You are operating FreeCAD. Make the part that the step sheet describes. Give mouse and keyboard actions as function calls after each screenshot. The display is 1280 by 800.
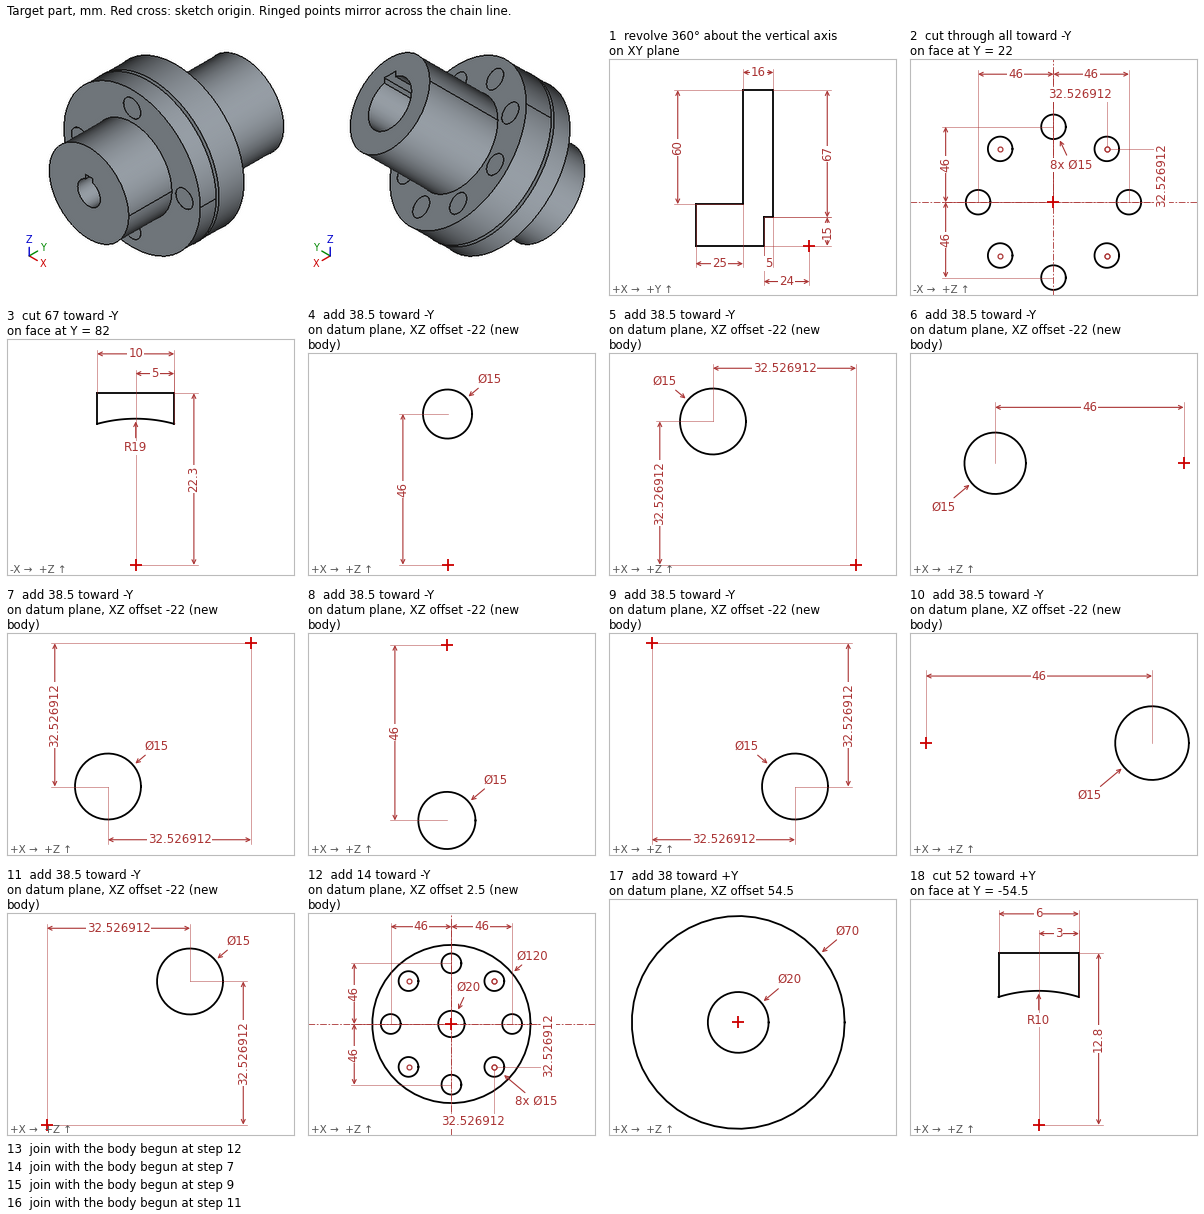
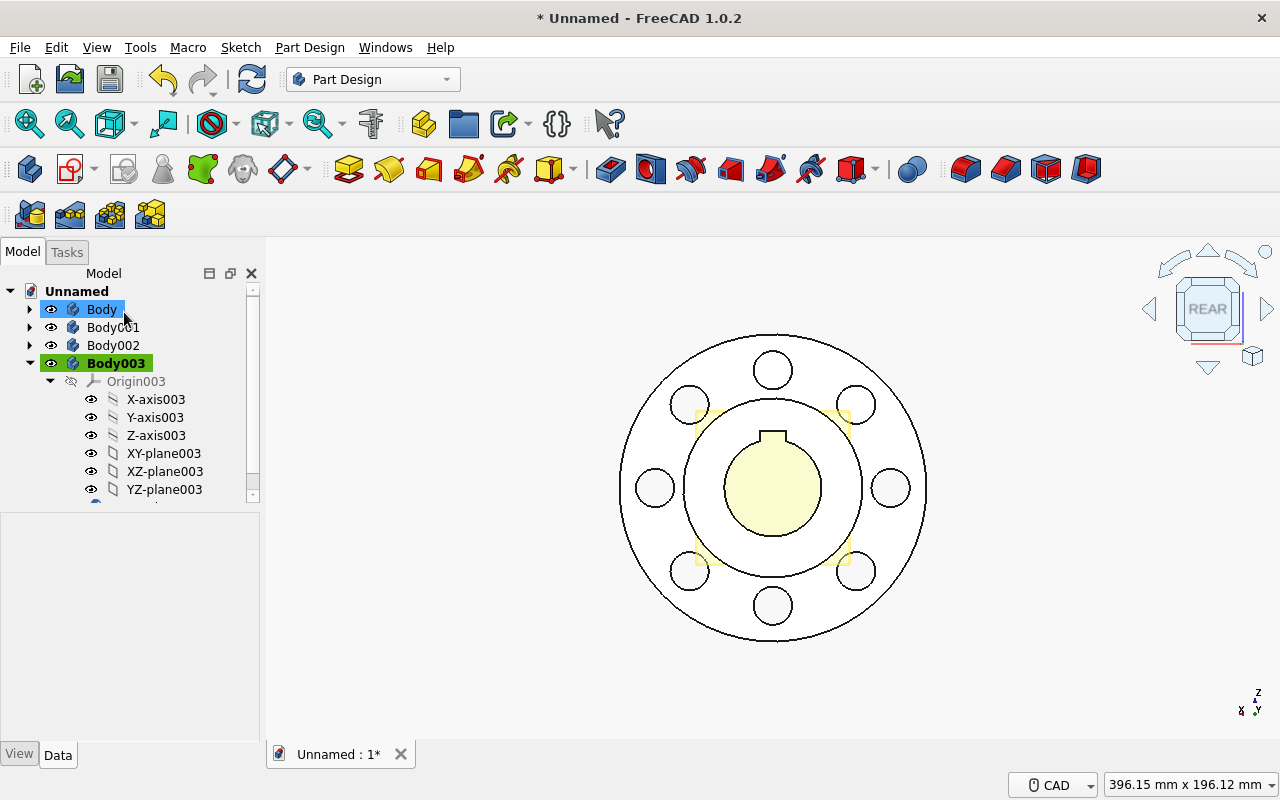
scroll(100, 395, down, 3)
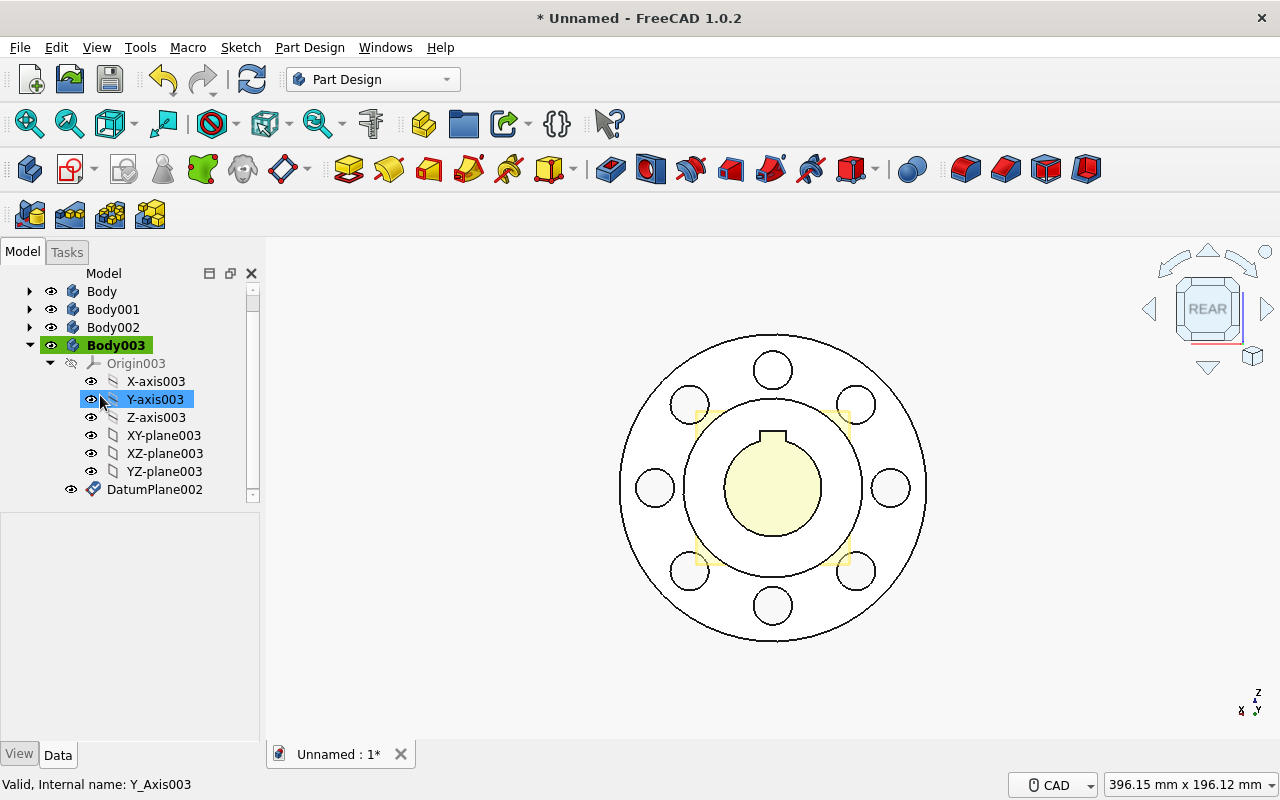
click(116, 489)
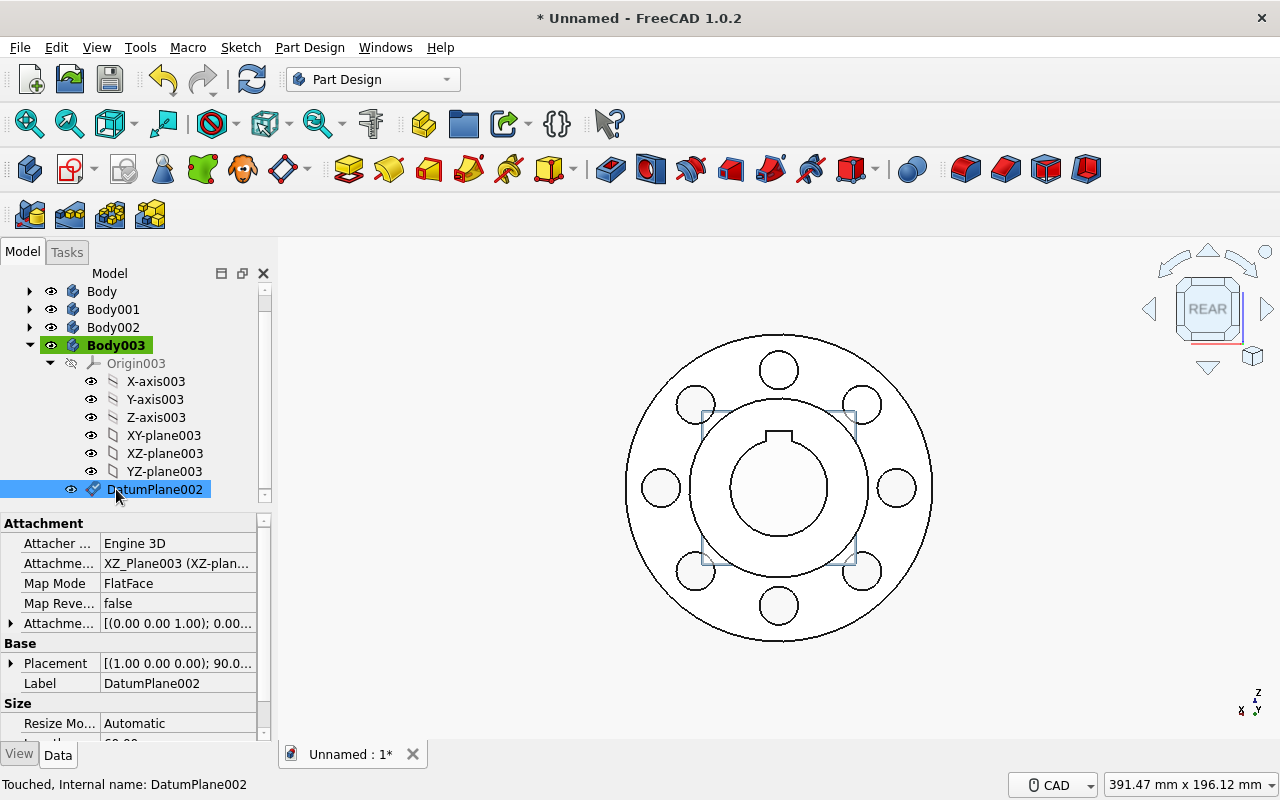
click(70, 170)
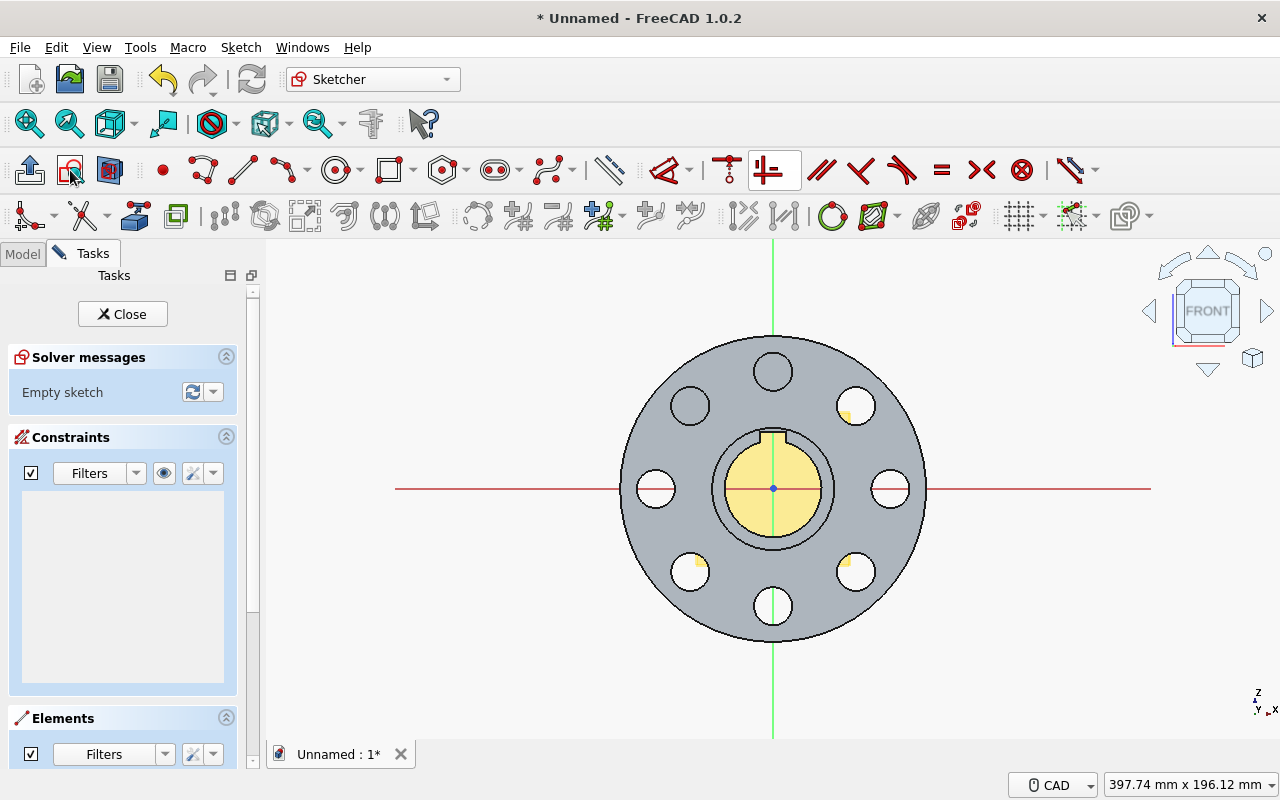
scroll(650, 489, up, 11)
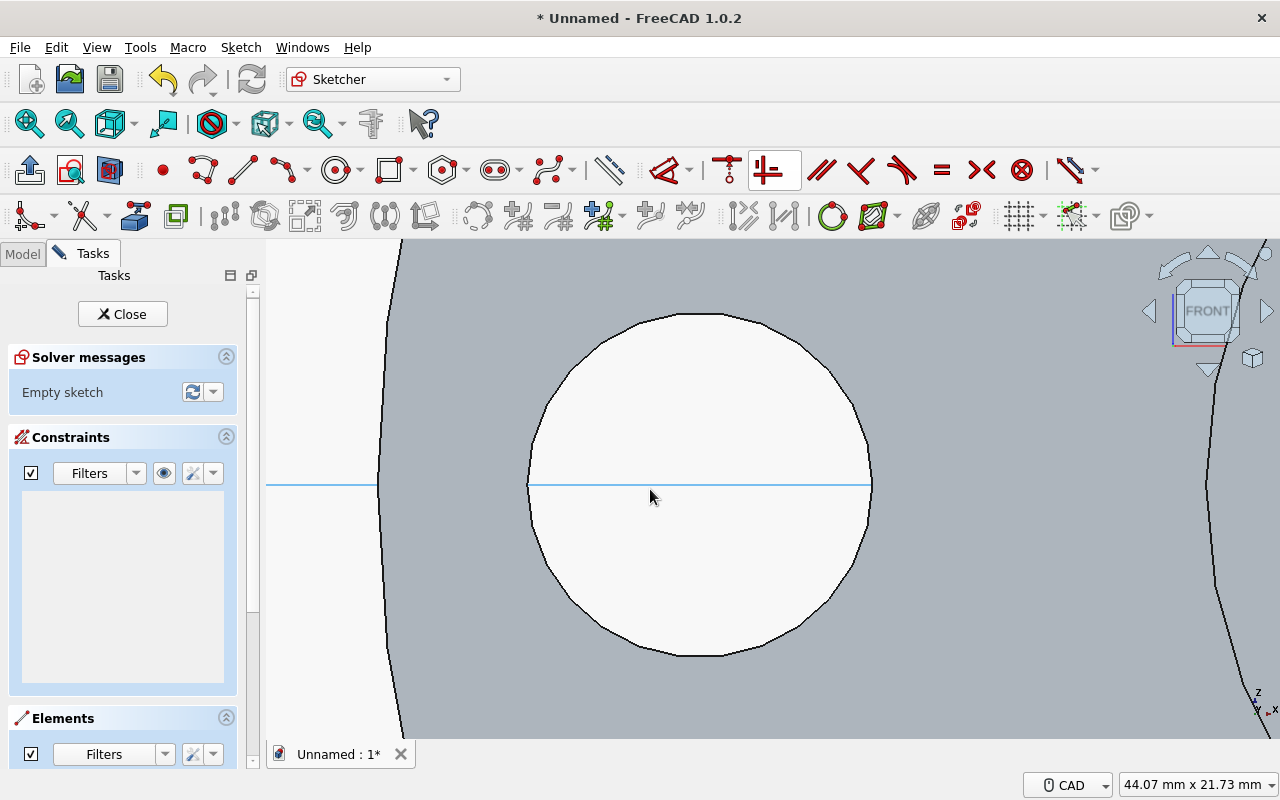
click(336, 170)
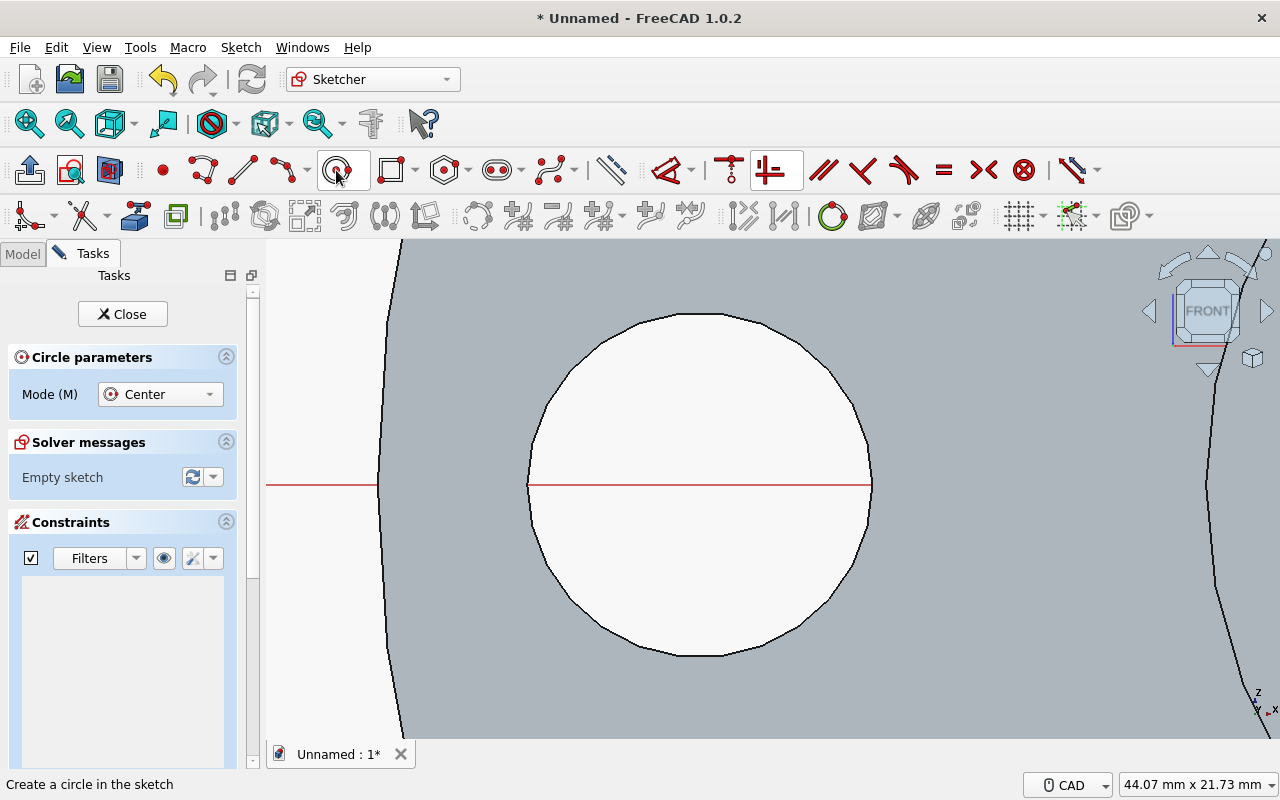
click(700, 485)
click(822, 363)
key(Escape)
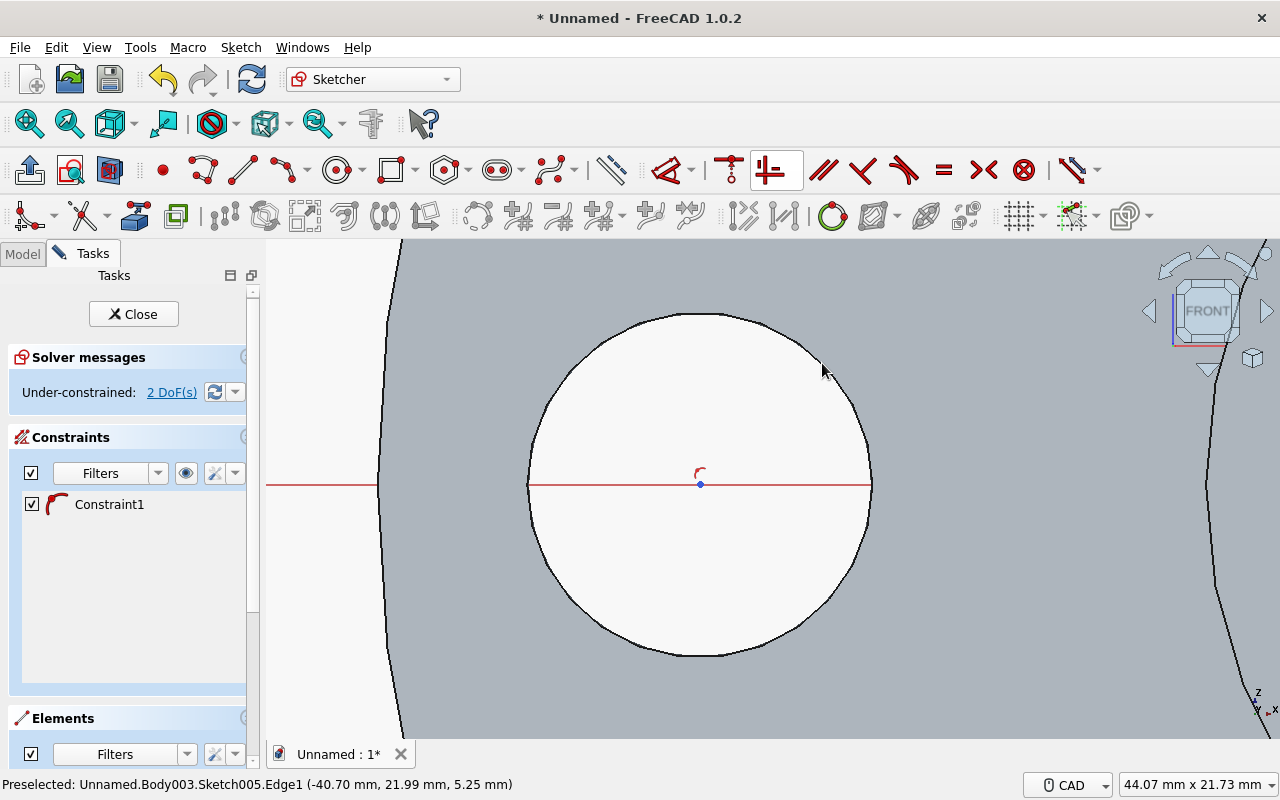
click(666, 170)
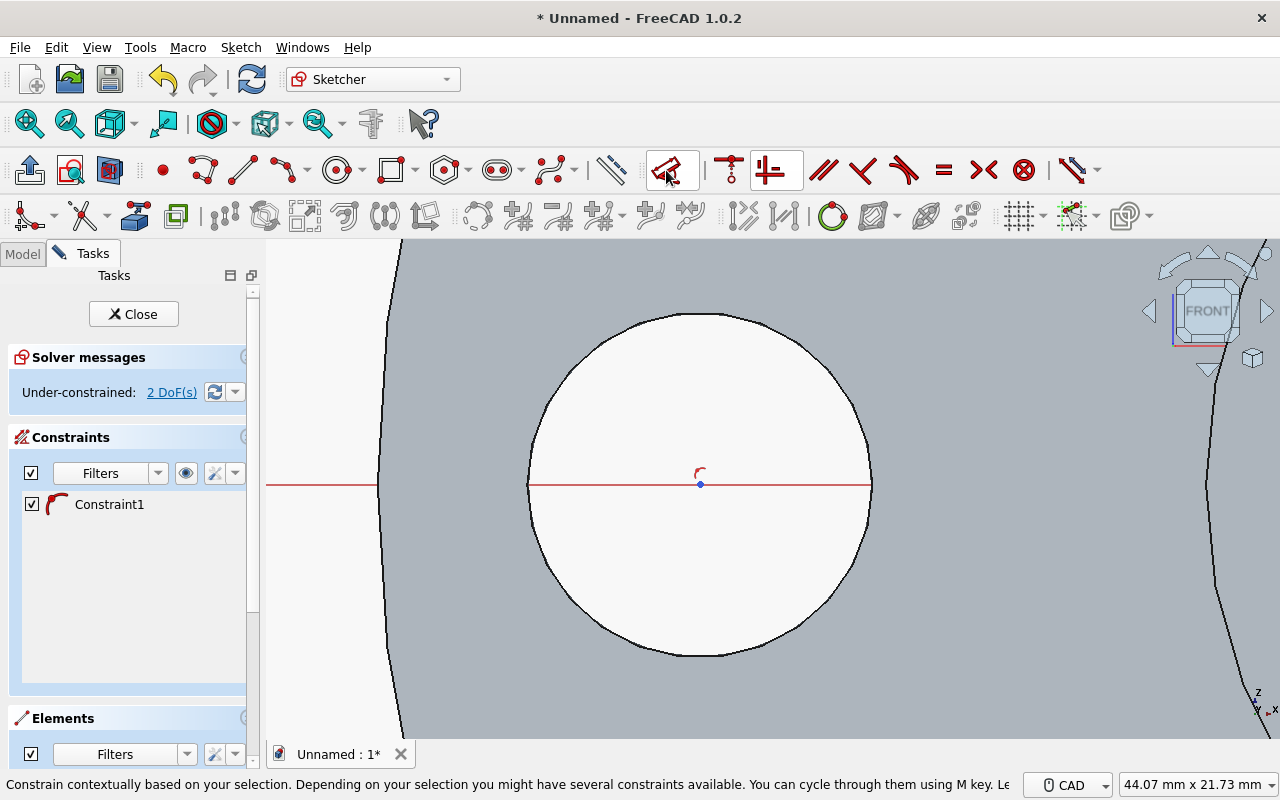
click(821, 363)
click(844, 340)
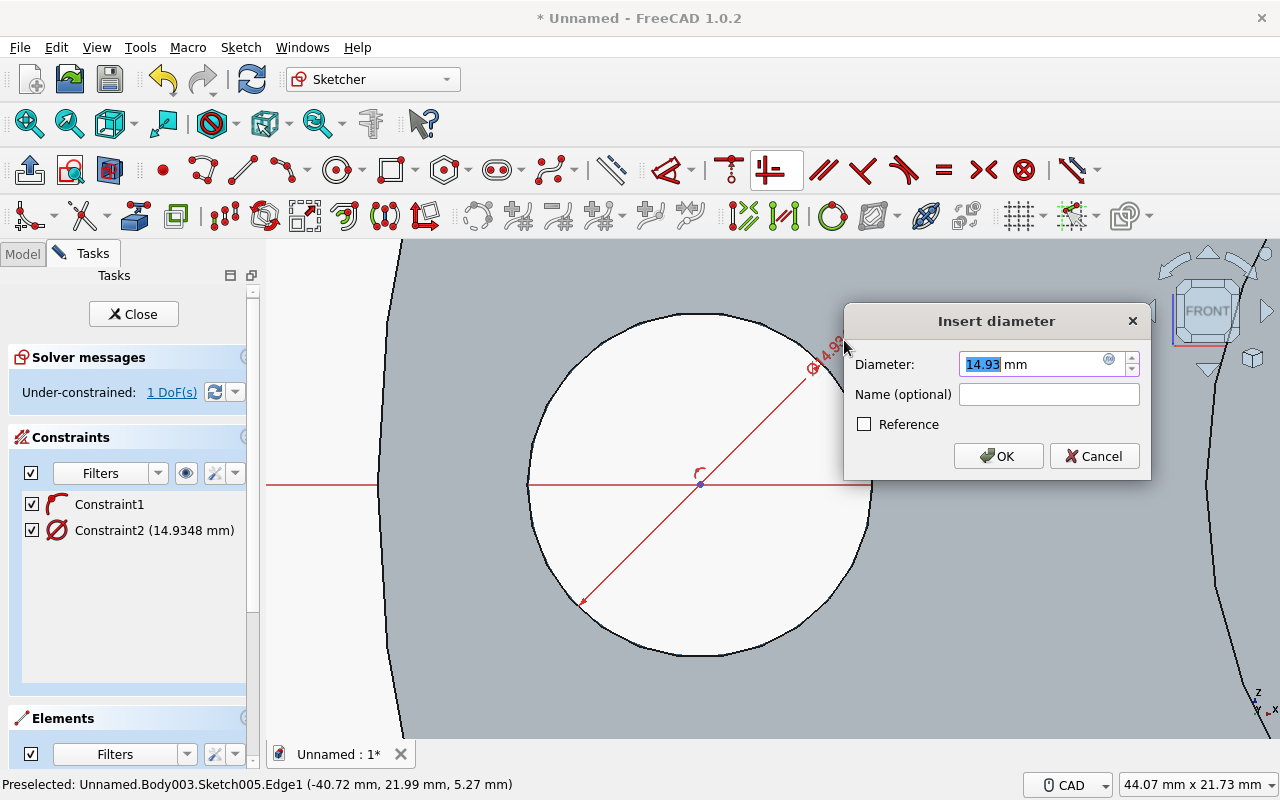
text(15)
key(Return)